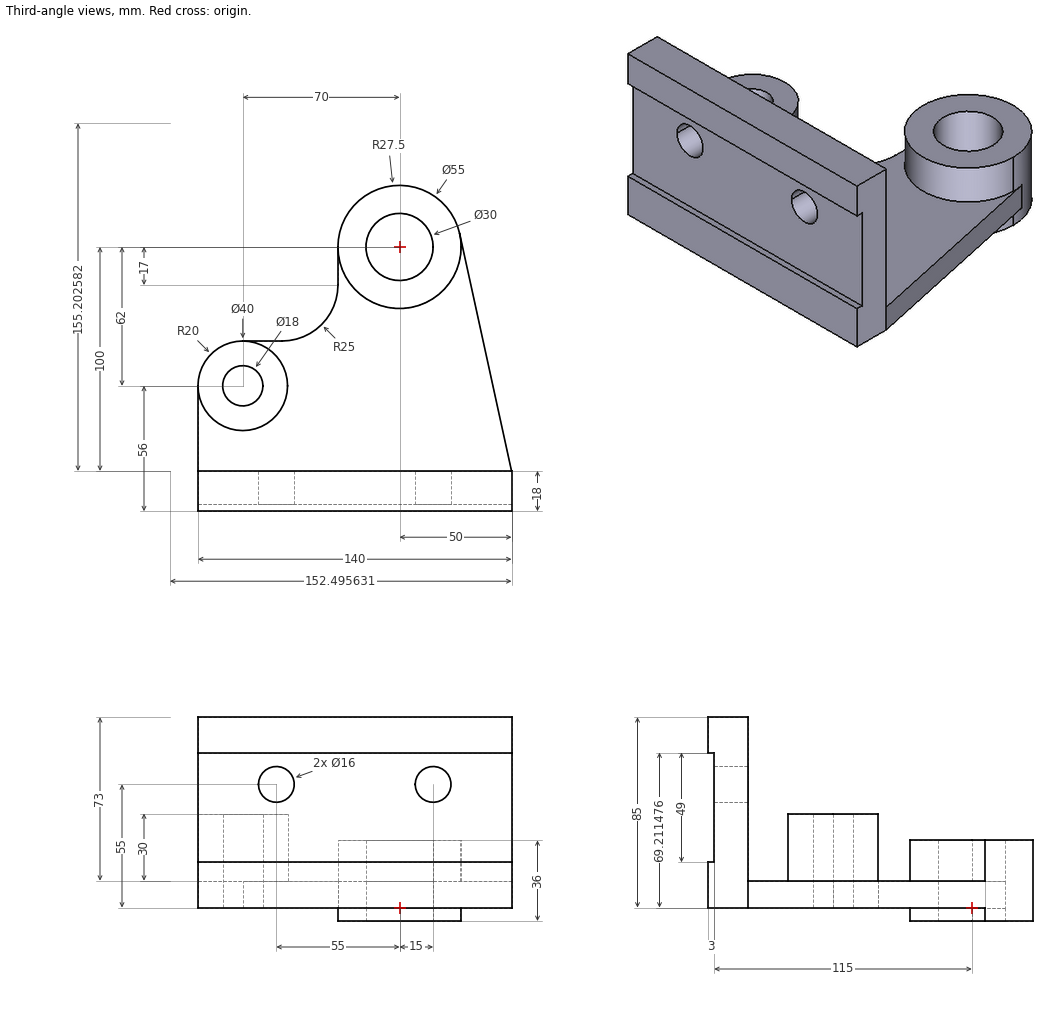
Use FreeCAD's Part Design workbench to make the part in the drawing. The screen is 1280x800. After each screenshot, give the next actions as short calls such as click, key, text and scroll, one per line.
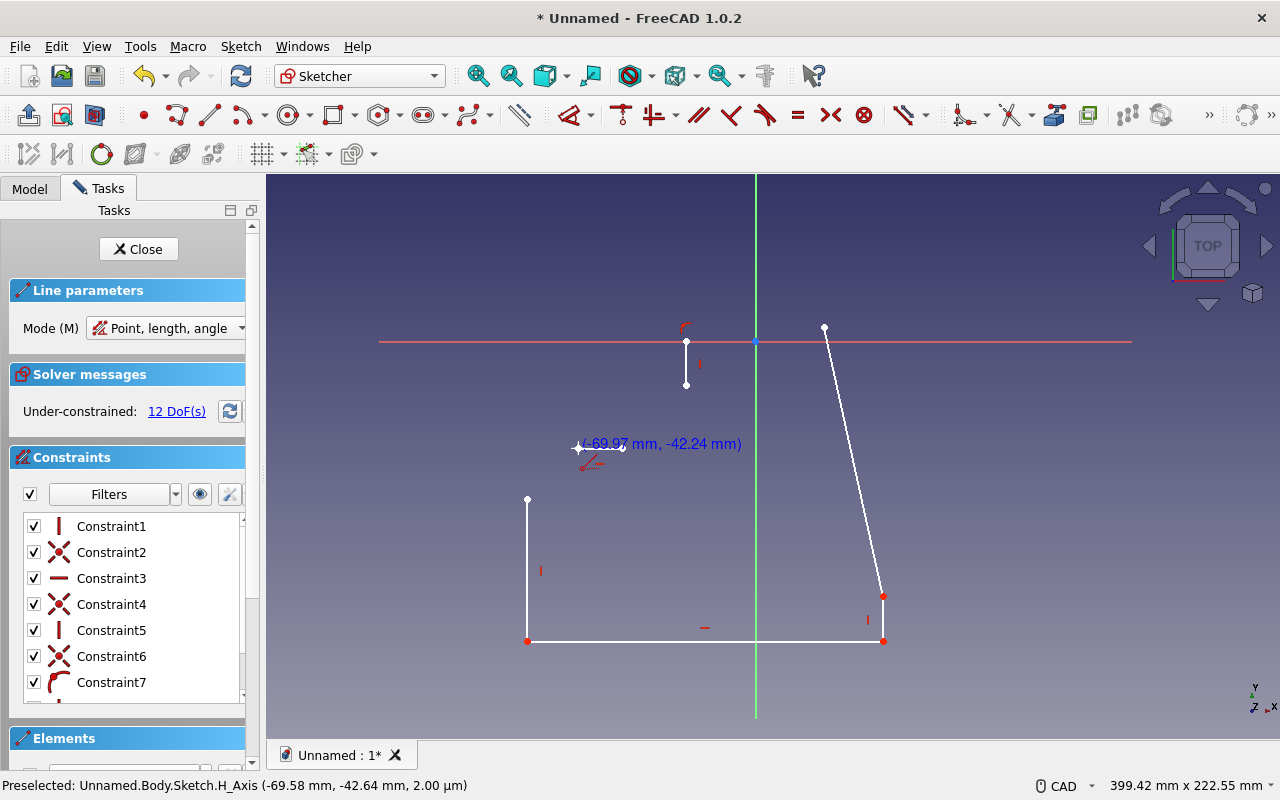
key(g)
key(3)
key(a)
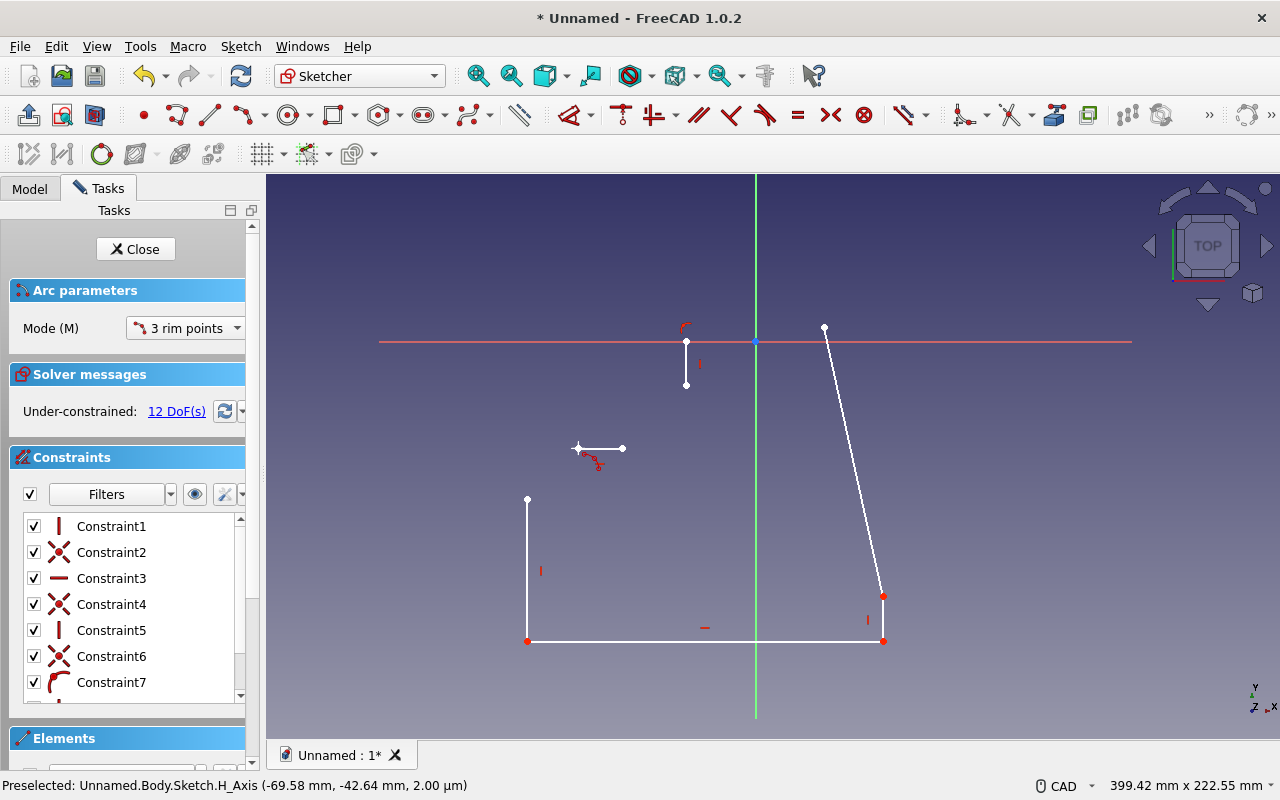
click(824, 328)
click(686, 342)
click(728, 277)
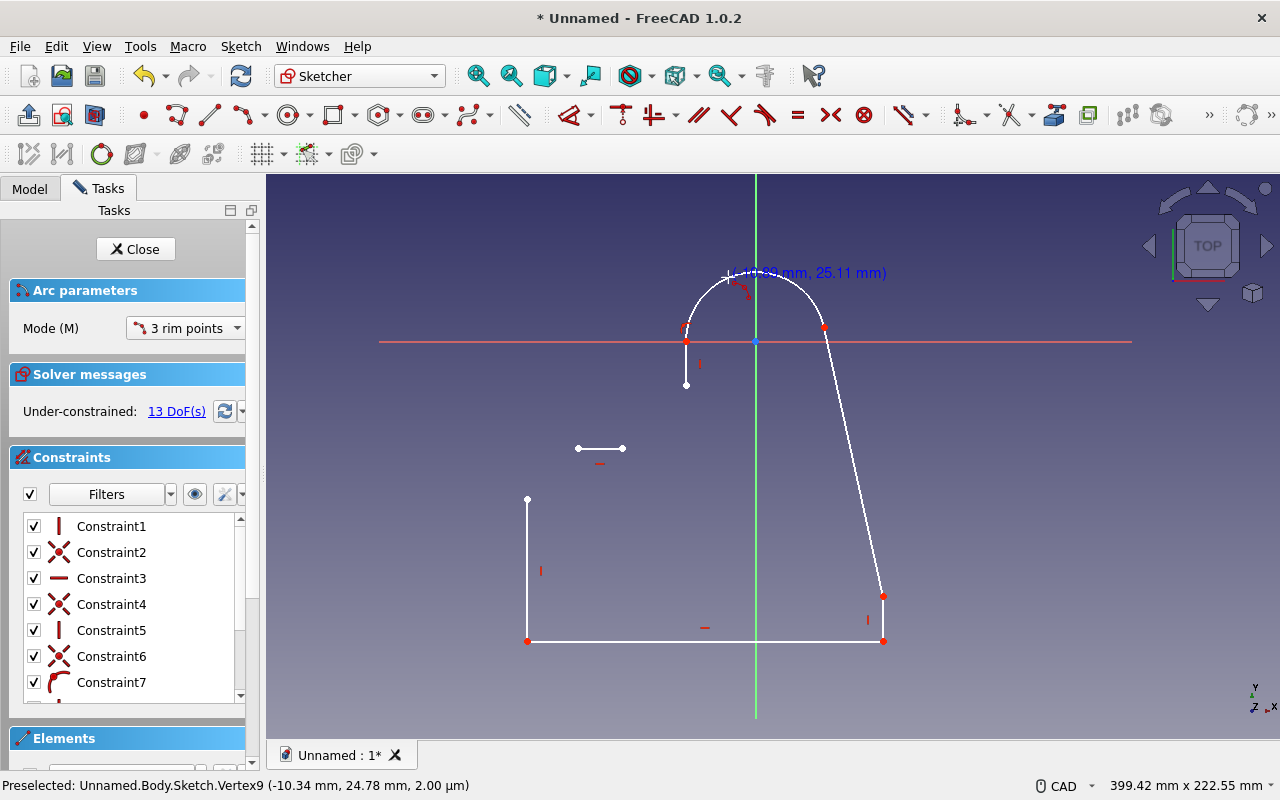
click(686, 386)
click(622, 449)
click(667, 430)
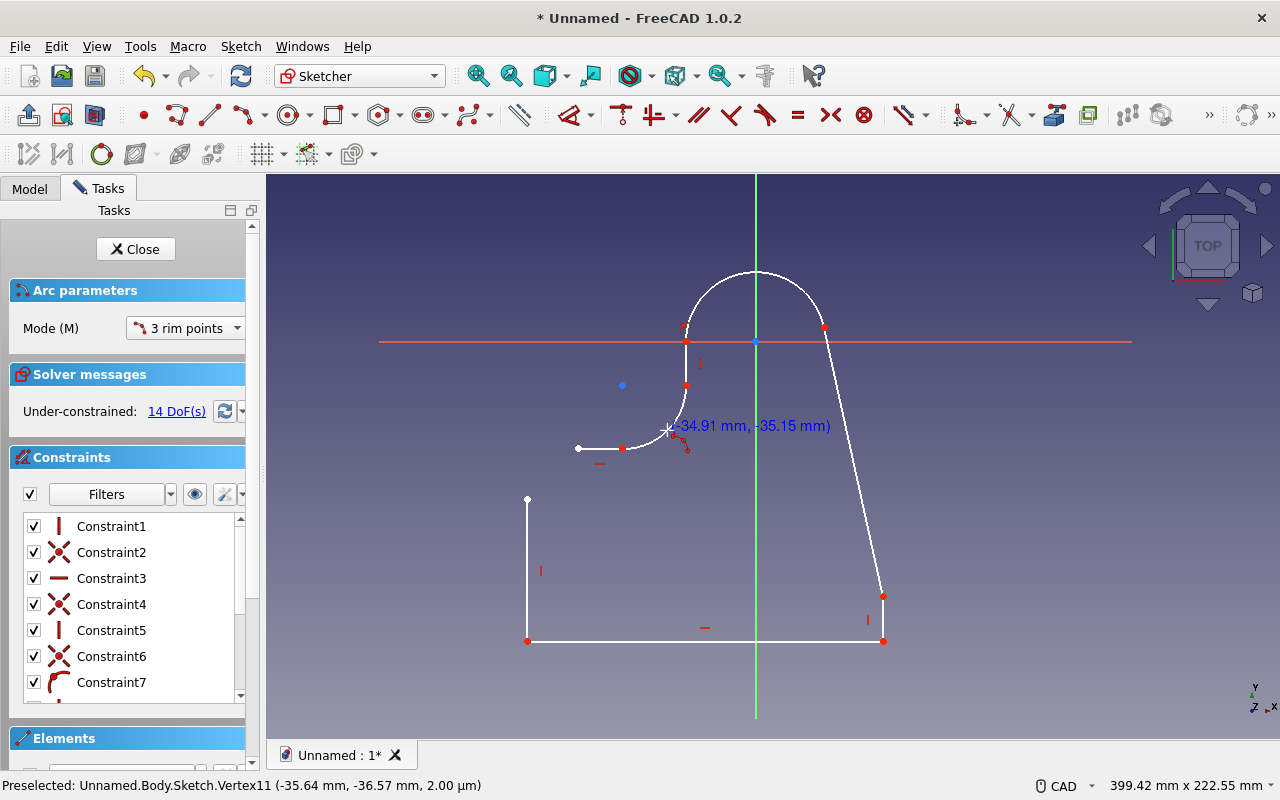
click(578, 449)
click(527, 500)
click(542, 463)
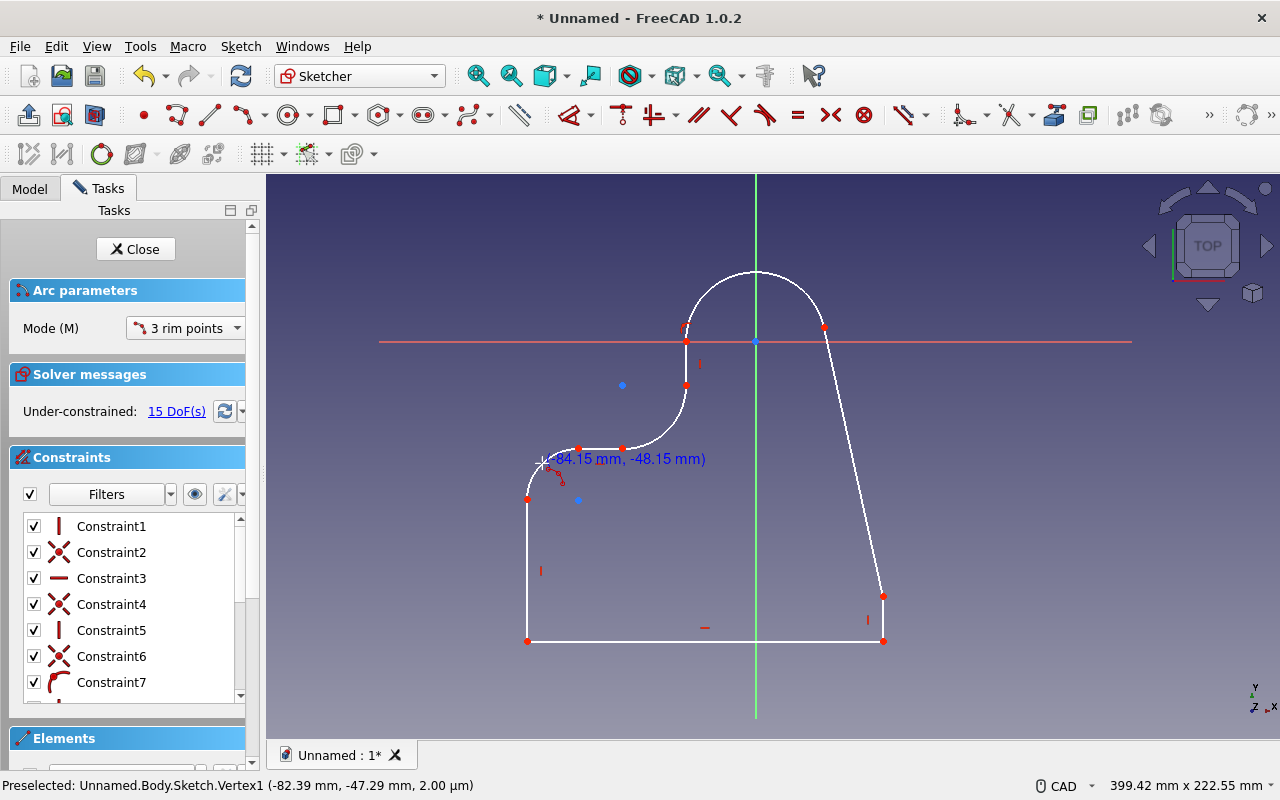
click(288, 116)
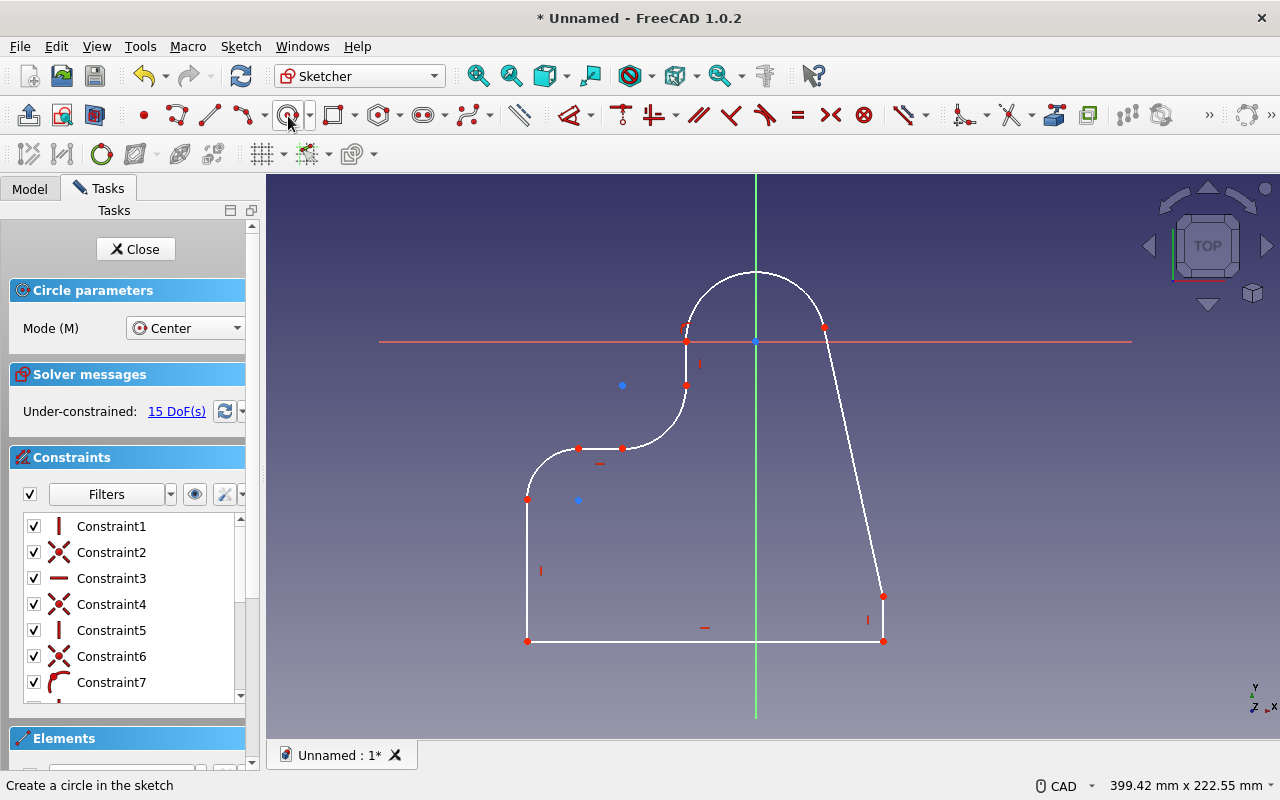
click(578, 499)
click(594, 483)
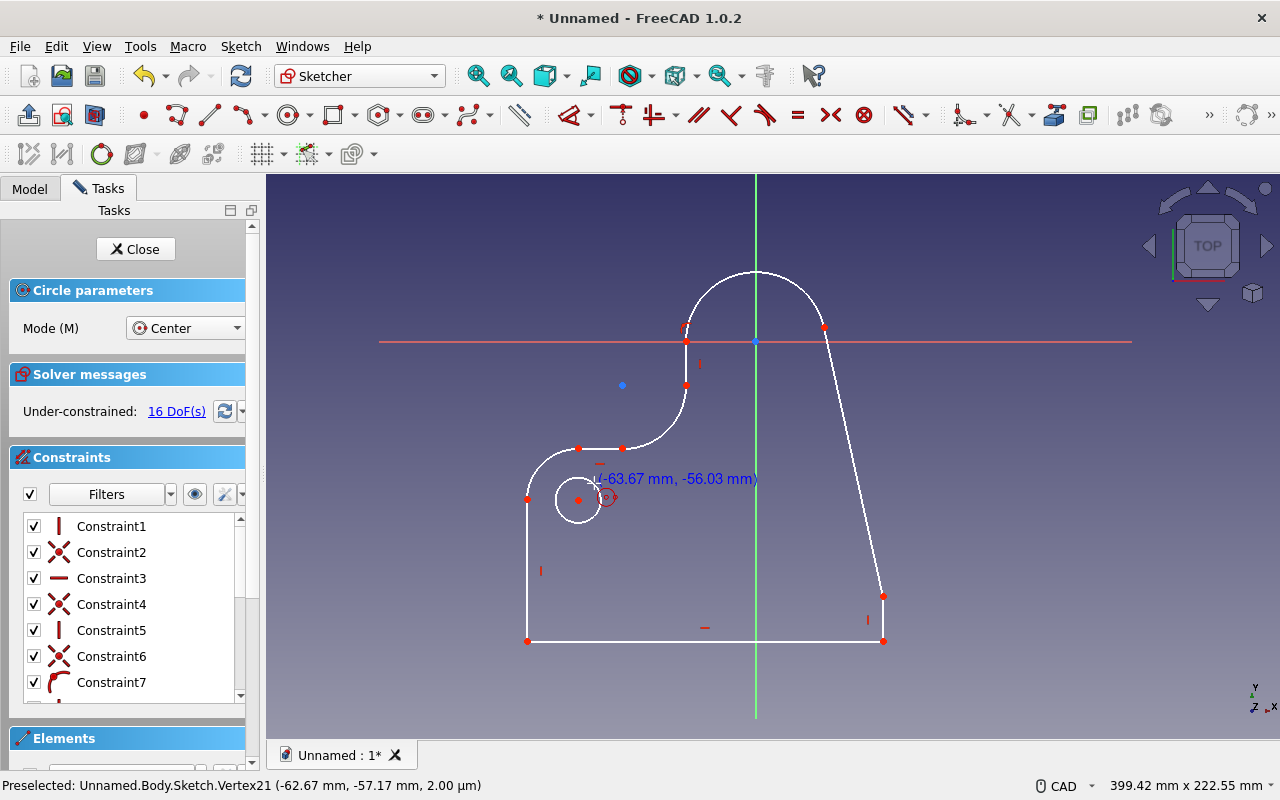
click(756, 342)
click(783, 315)
key(Escape)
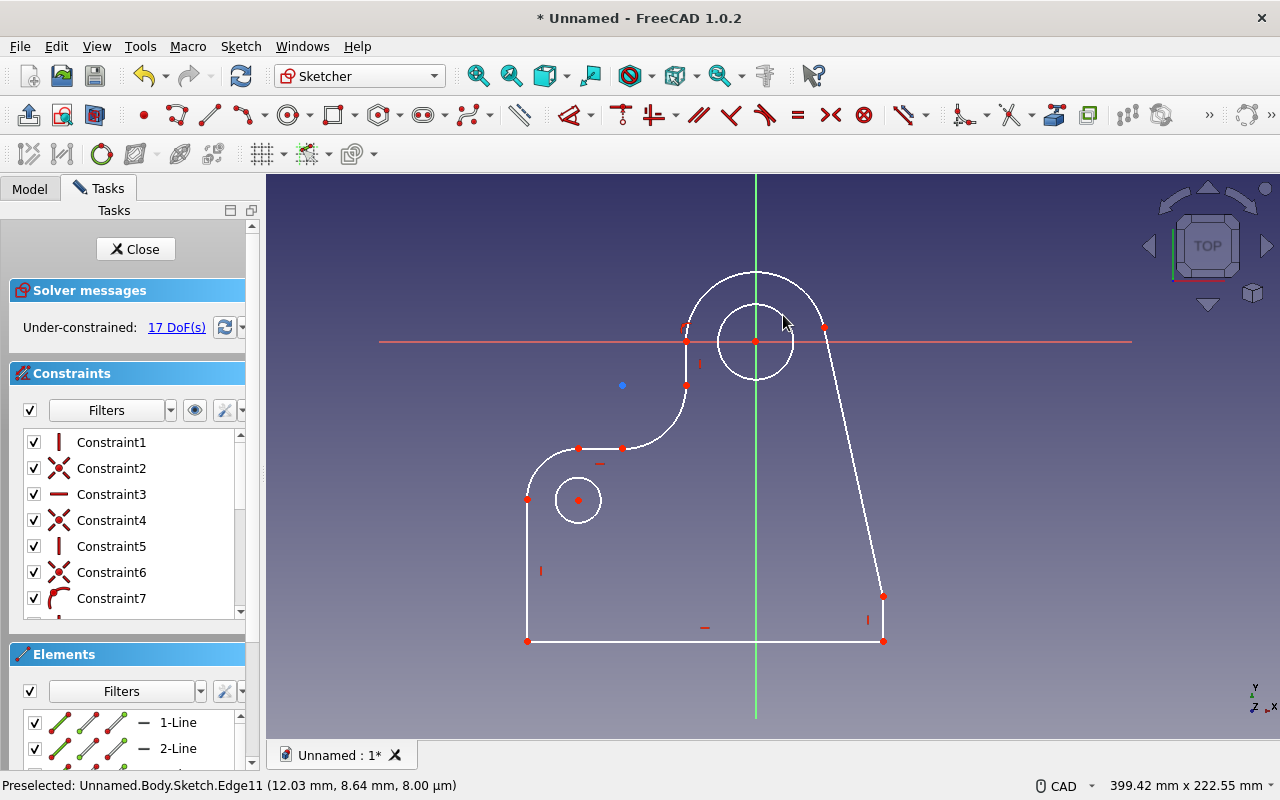
click(527, 543)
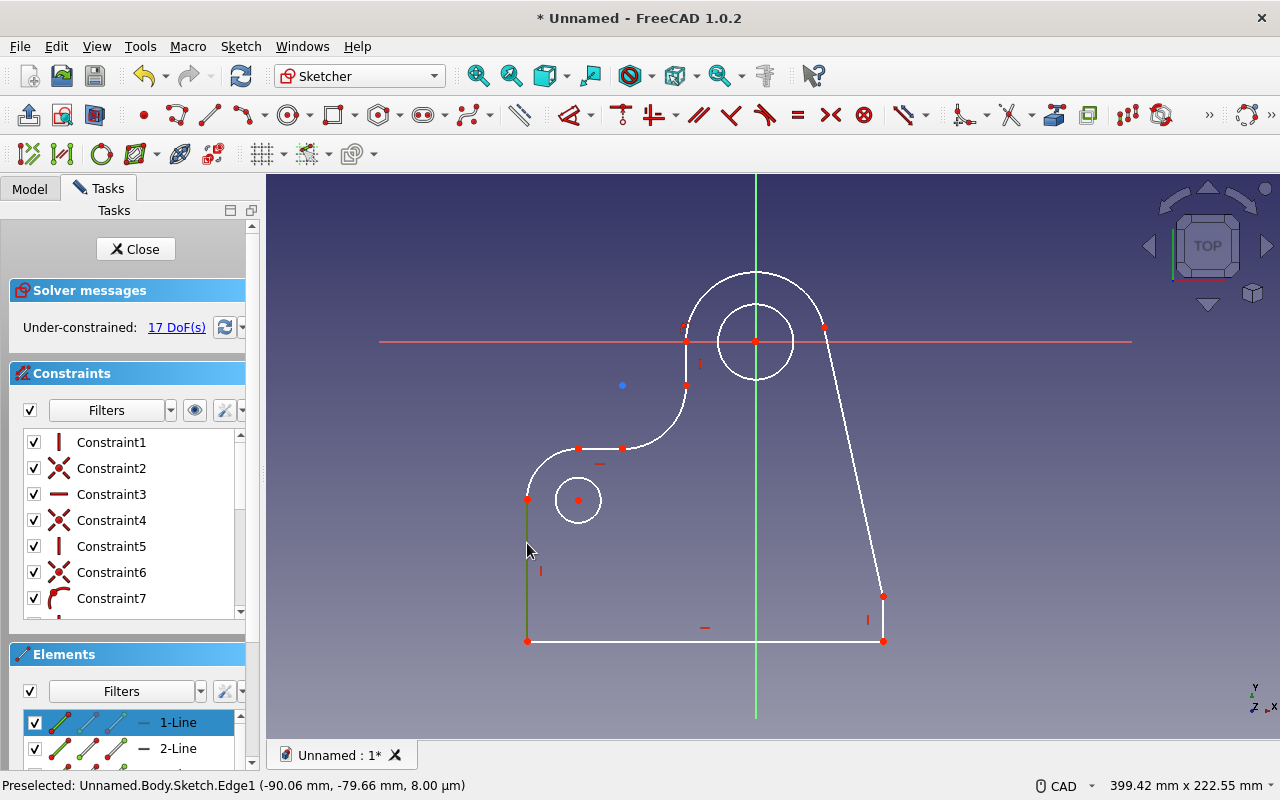
click(555, 455)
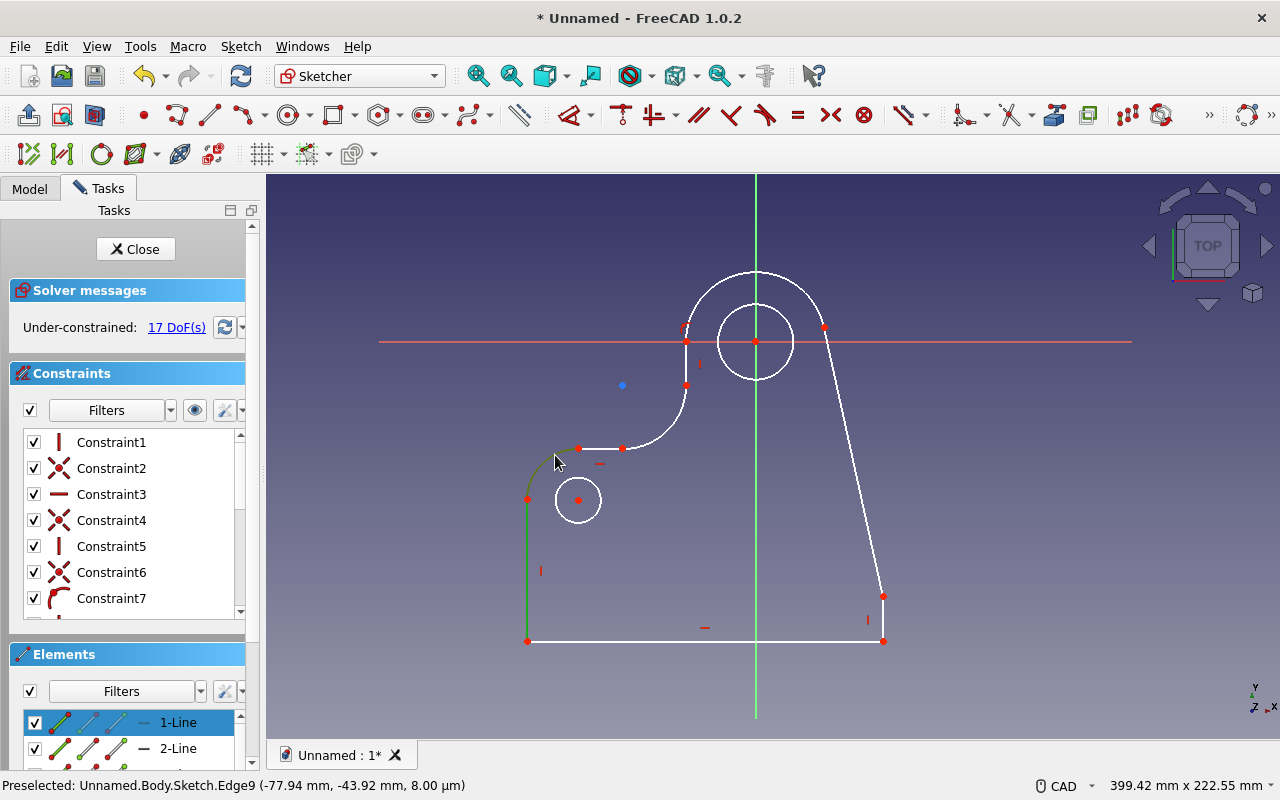
click(765, 116)